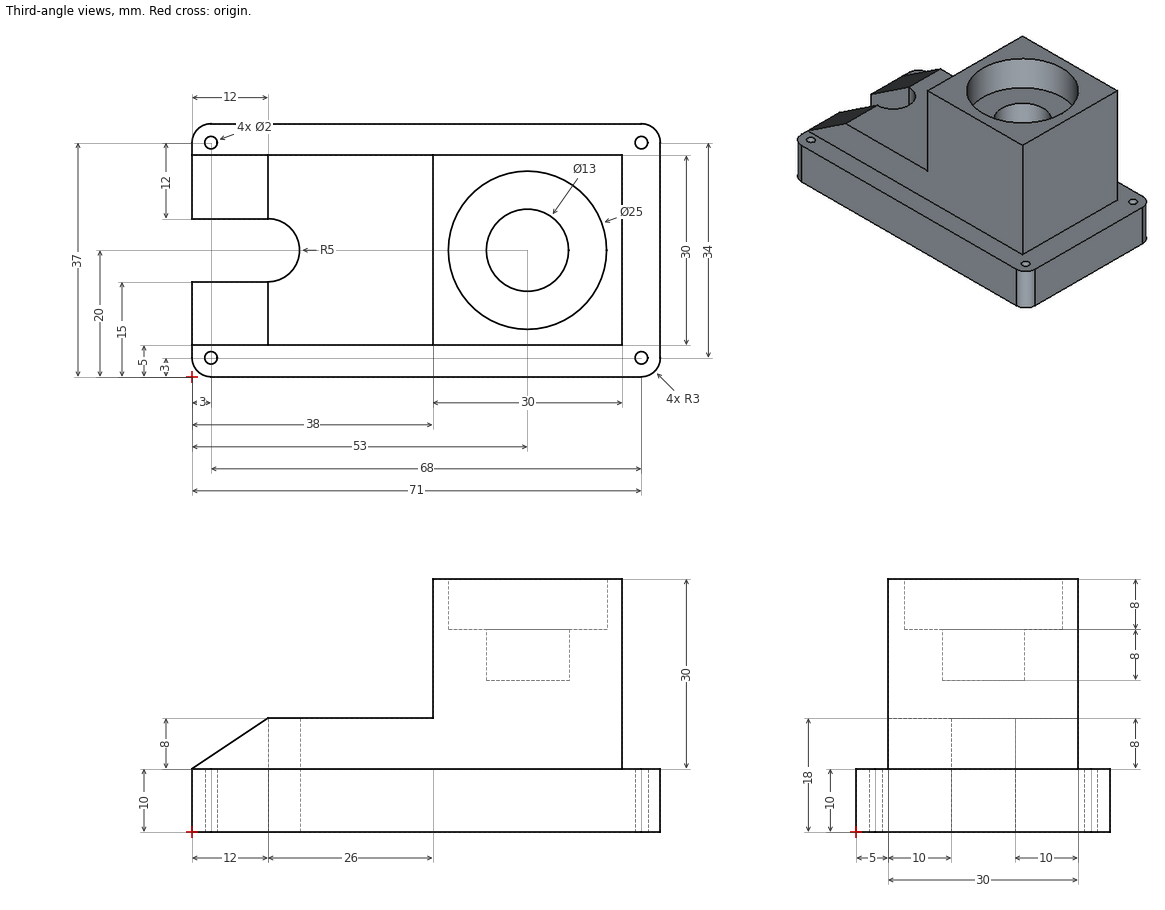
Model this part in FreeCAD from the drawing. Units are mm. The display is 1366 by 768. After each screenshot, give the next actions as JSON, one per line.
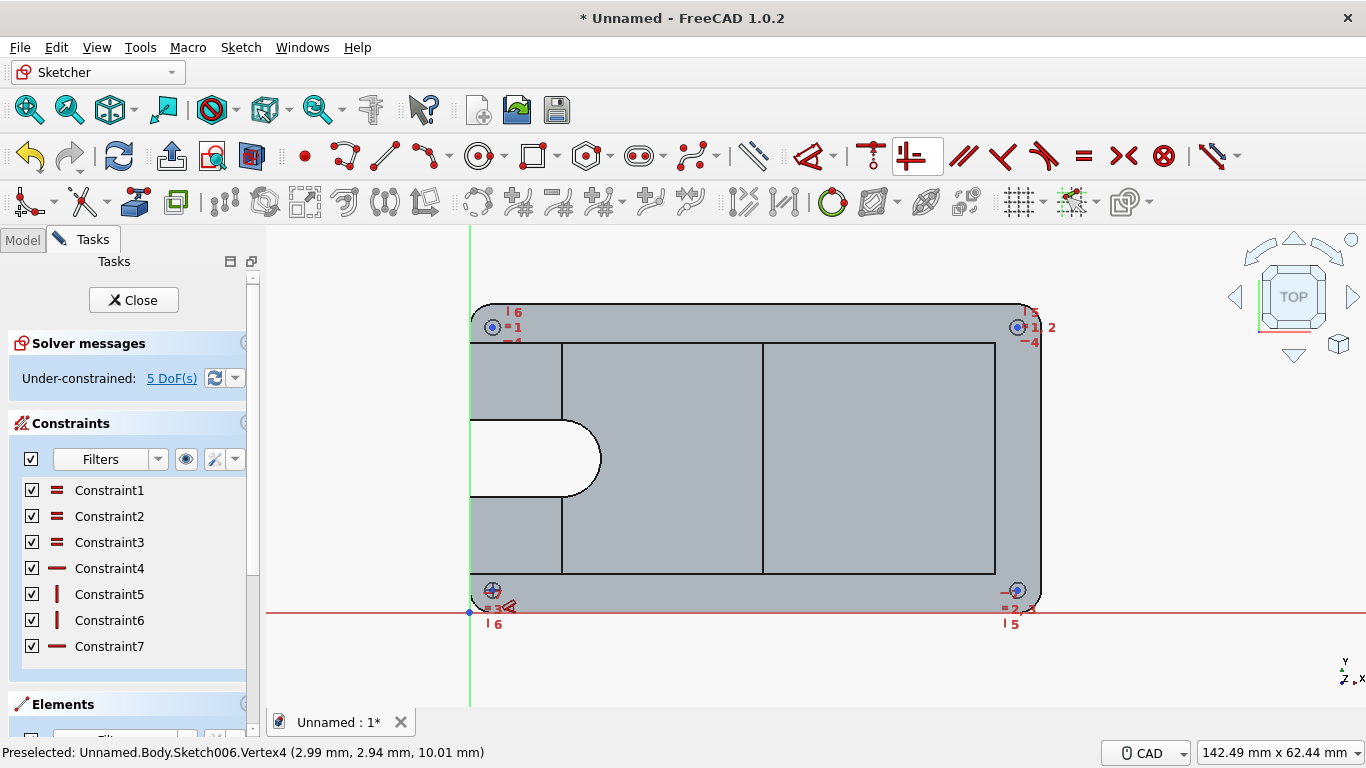
{"action": "scroll", "coordinate": [487, 322], "scroll_direction": "up", "scroll_amount": 5}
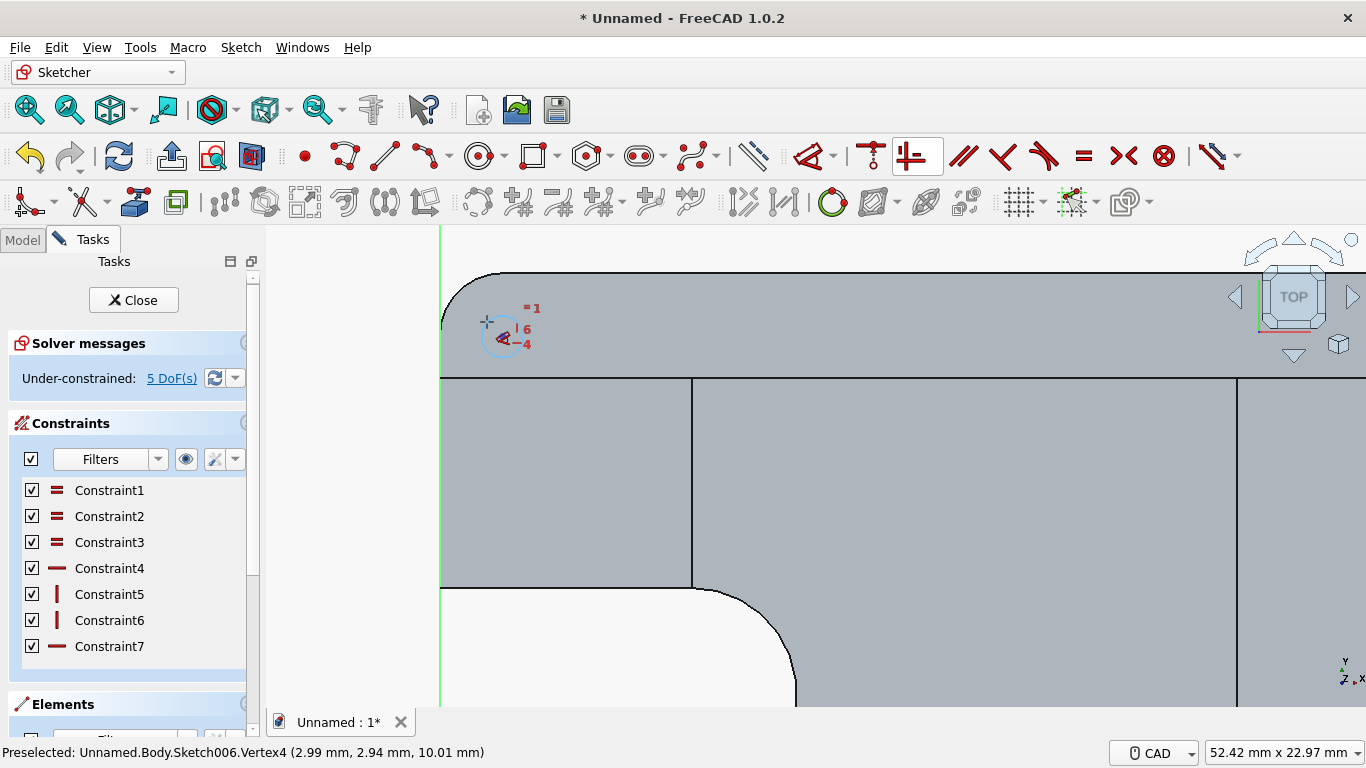
{"action": "left_click", "coordinate": [488, 322]}
{"action": "left_click", "coordinate": [466, 299]}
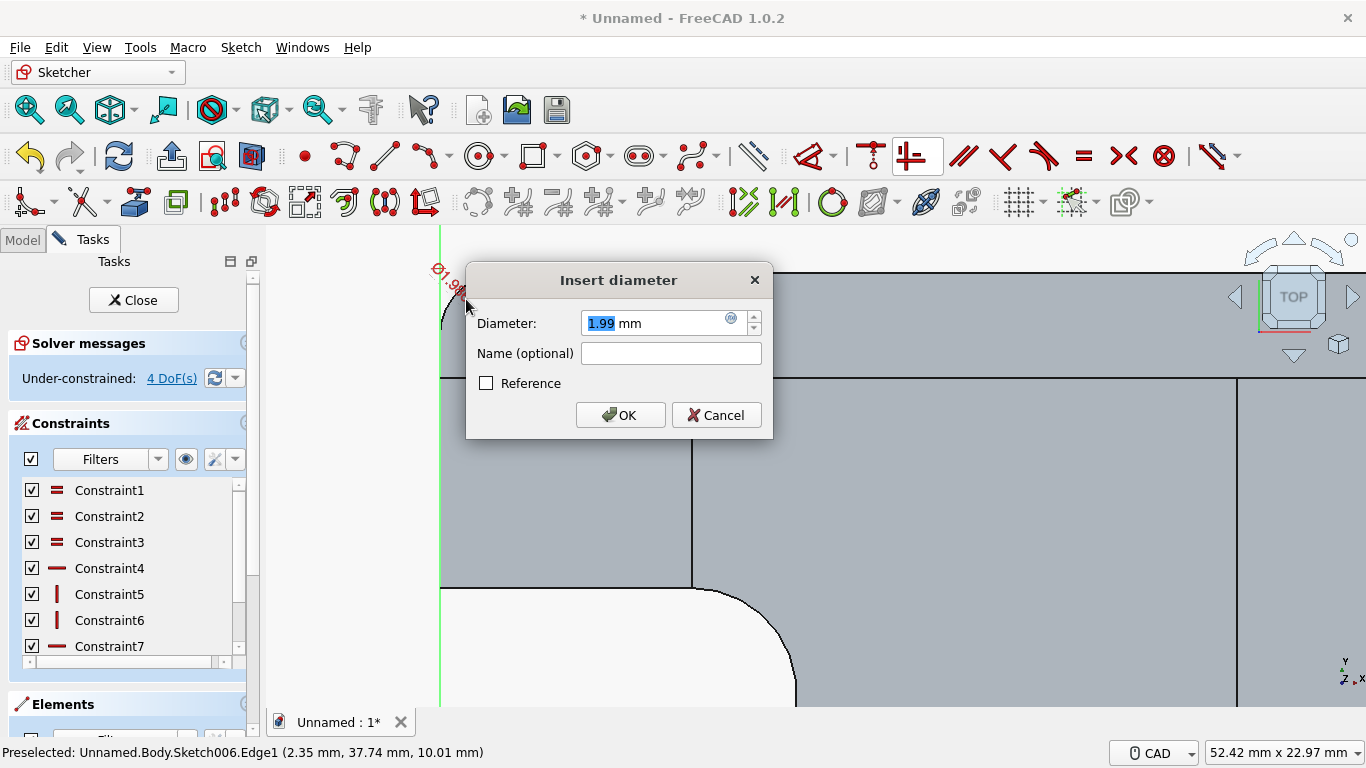
{"action": "type", "text": "2"}
{"action": "key", "text": "Return"}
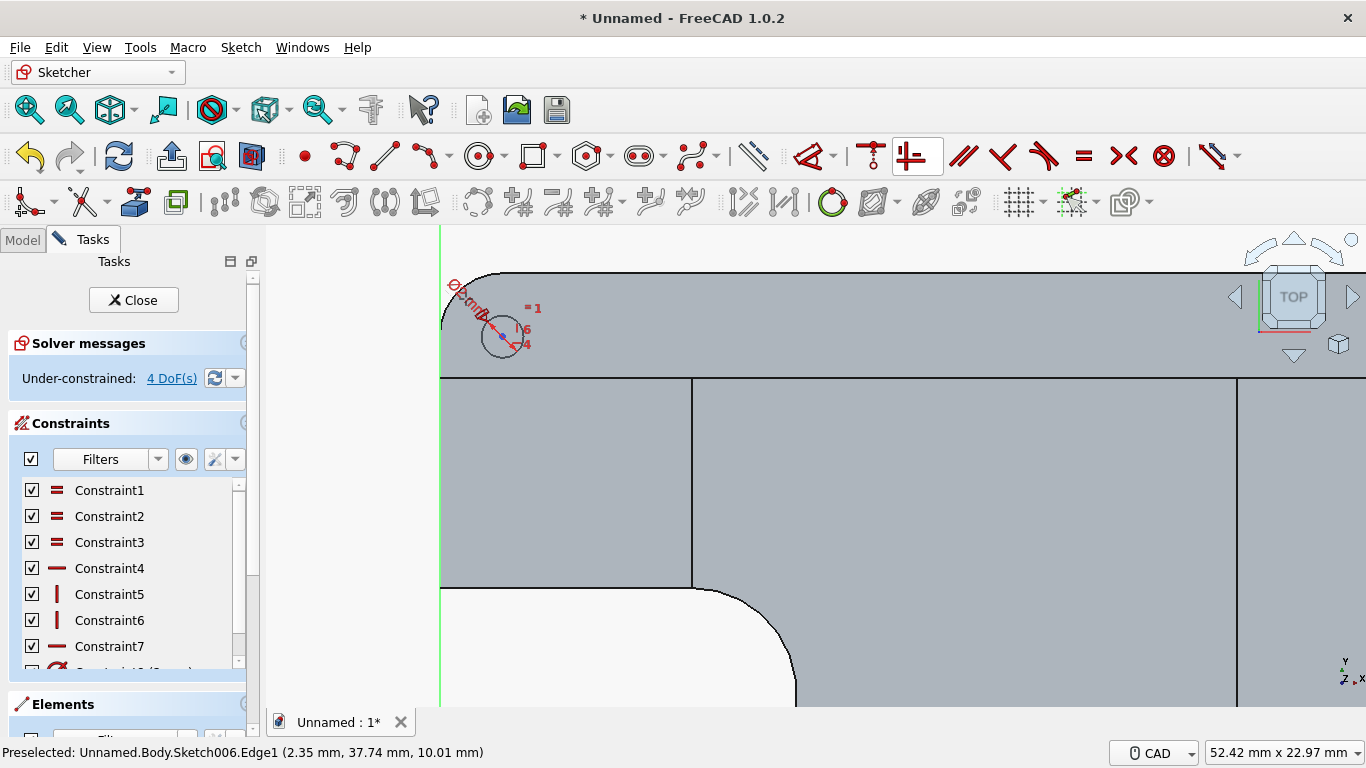
{"action": "left_click", "coordinate": [503, 337]}
{"action": "left_click", "coordinate": [471, 279]}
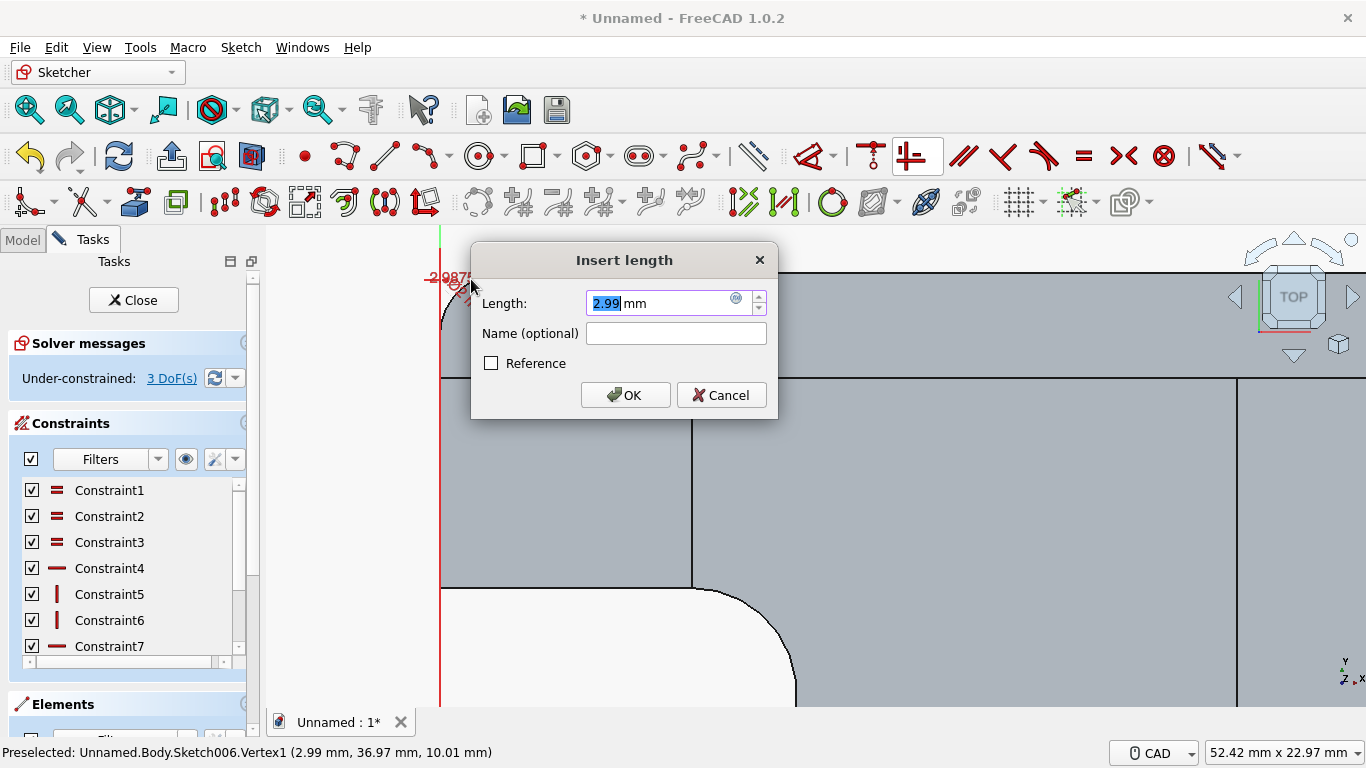
{"action": "type", "text": "3"}
{"action": "key", "text": "Return"}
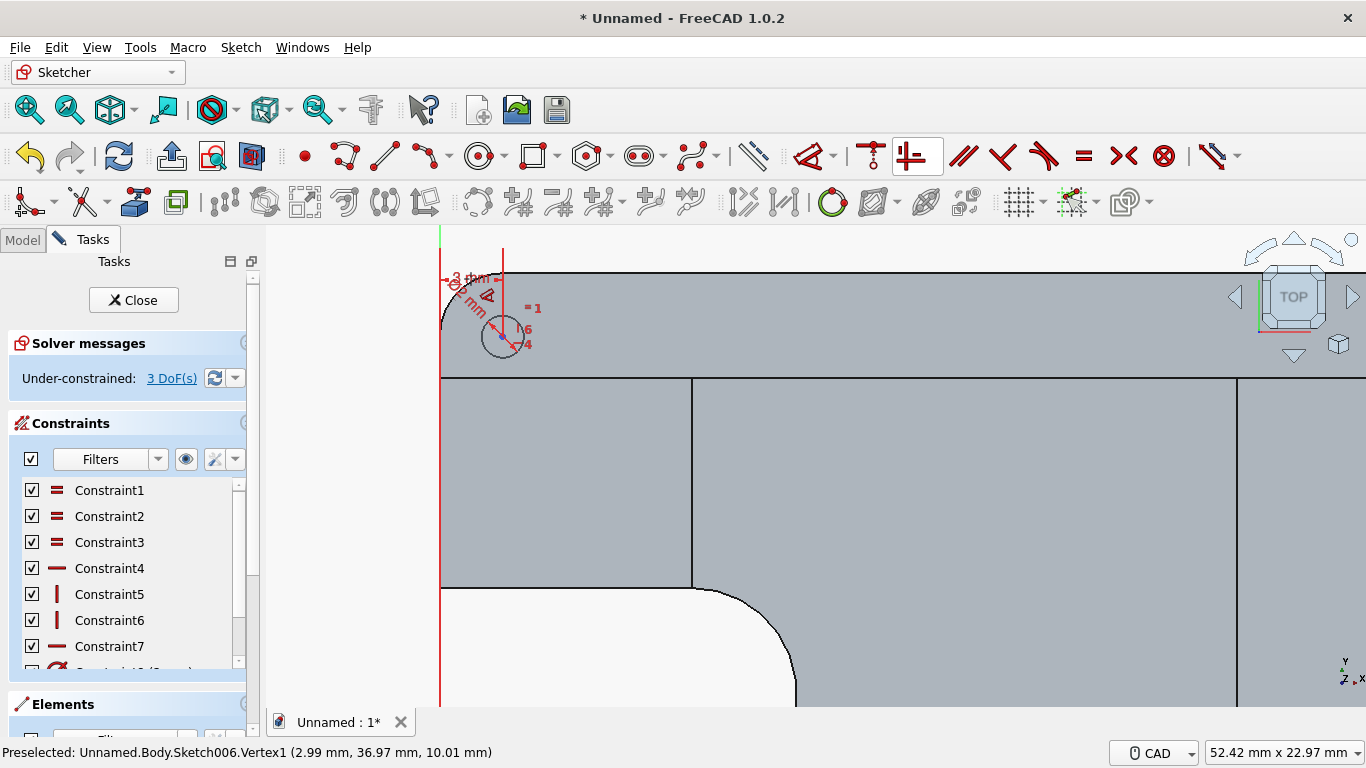
{"action": "scroll", "coordinate": [487, 322], "scroll_direction": "down", "scroll_amount": 5}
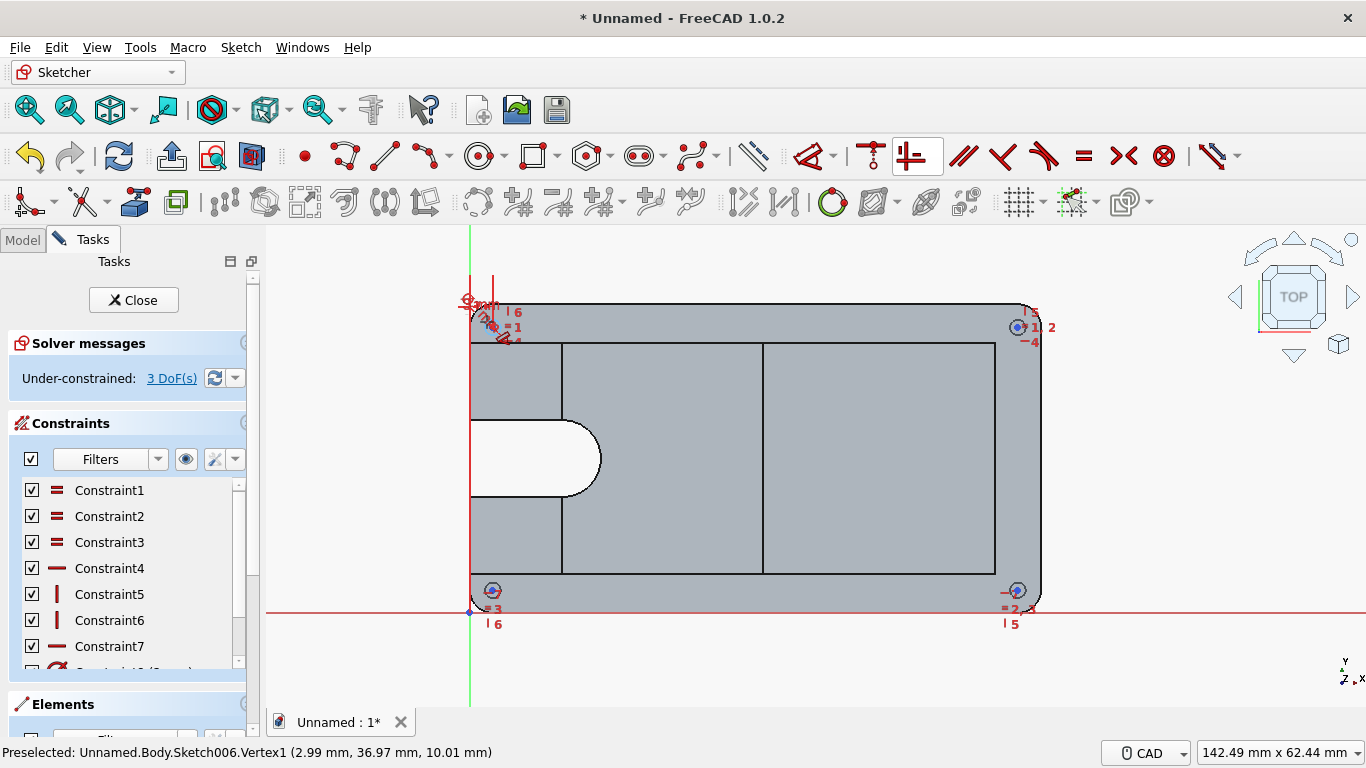
{"action": "scroll", "coordinate": [1018, 590], "scroll_direction": "up", "scroll_amount": 3}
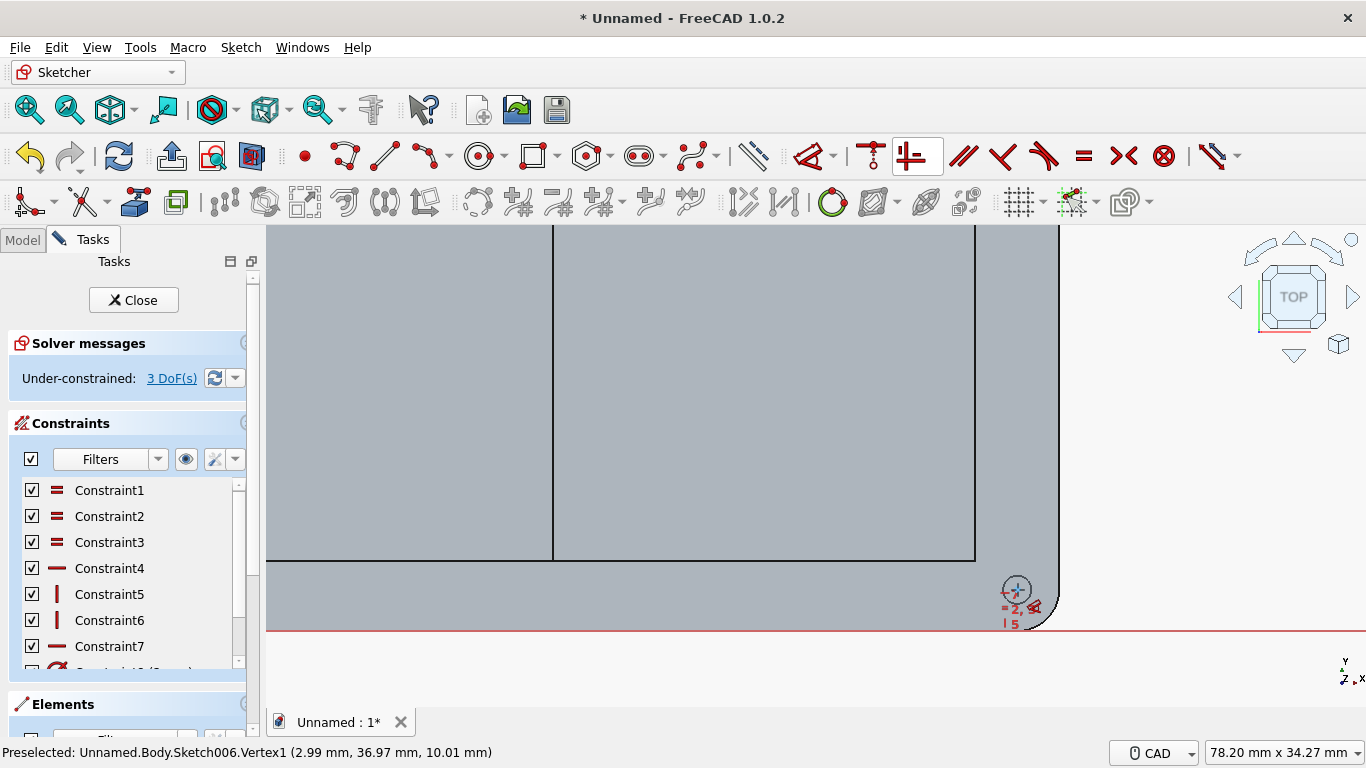
{"action": "left_click", "coordinate": [1017, 590]}
{"action": "left_click", "coordinate": [1051, 611]}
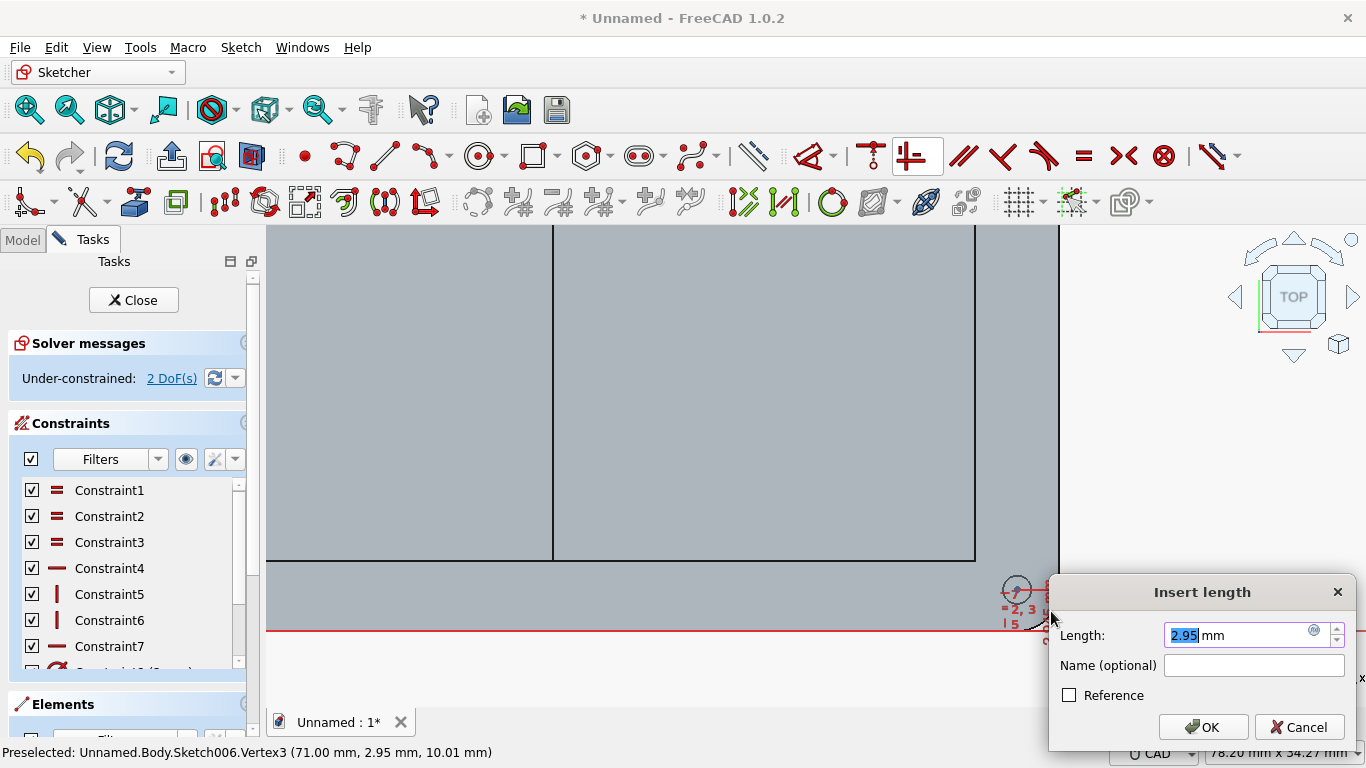
{"action": "type", "text": "3"}
{"action": "key", "text": "Return"}